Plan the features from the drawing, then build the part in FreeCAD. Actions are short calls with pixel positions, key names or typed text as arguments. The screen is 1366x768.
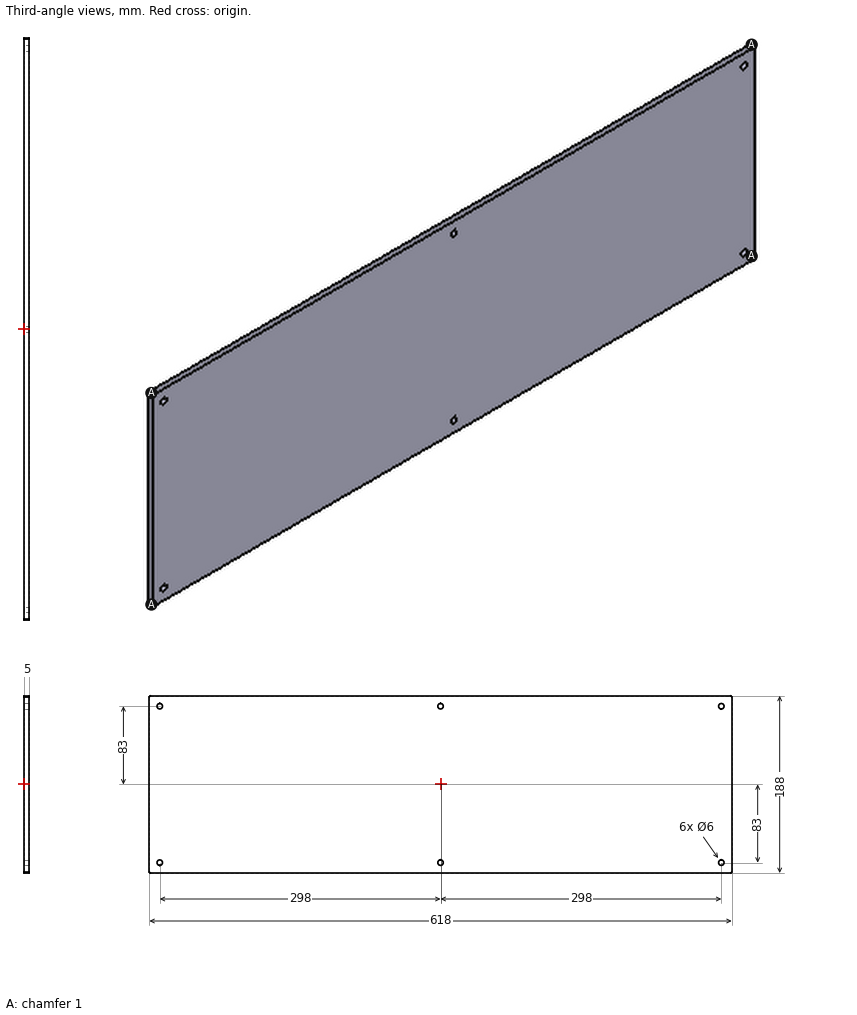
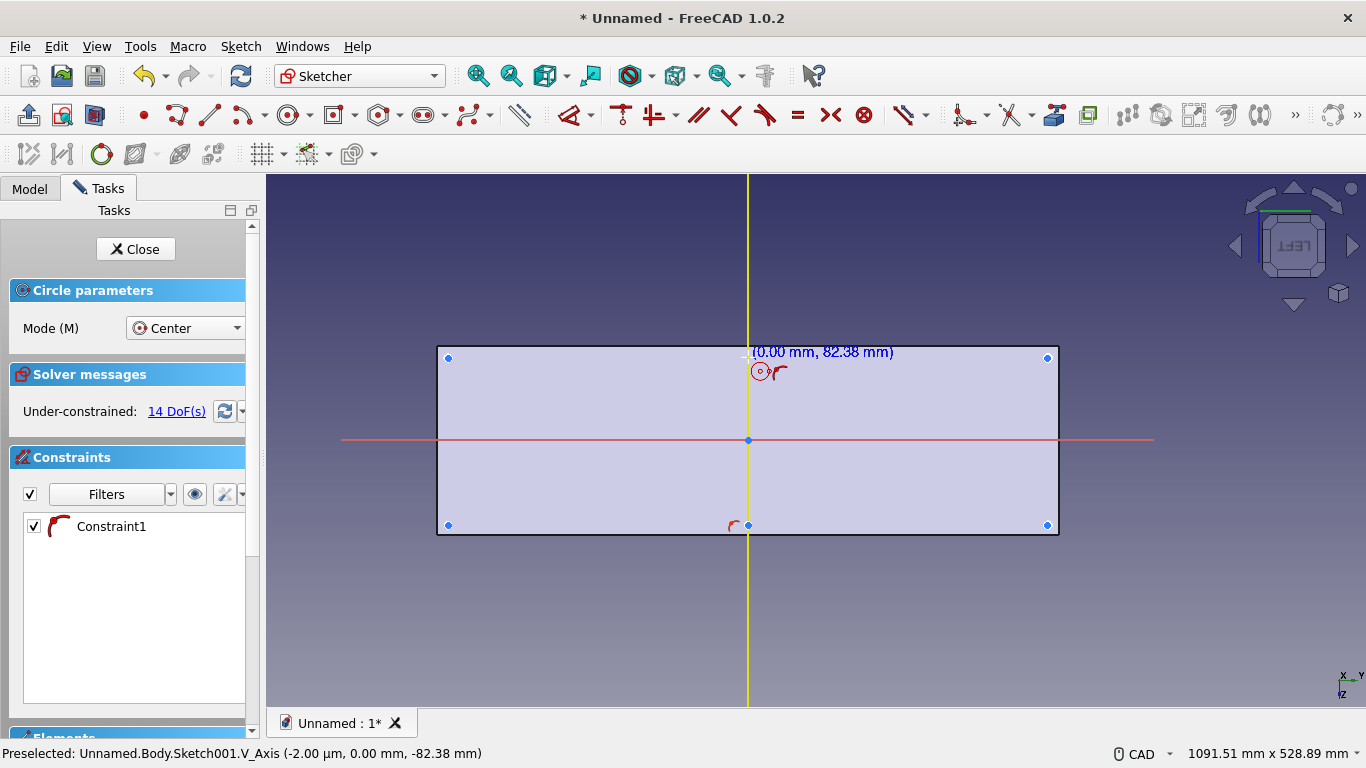
click(748, 357)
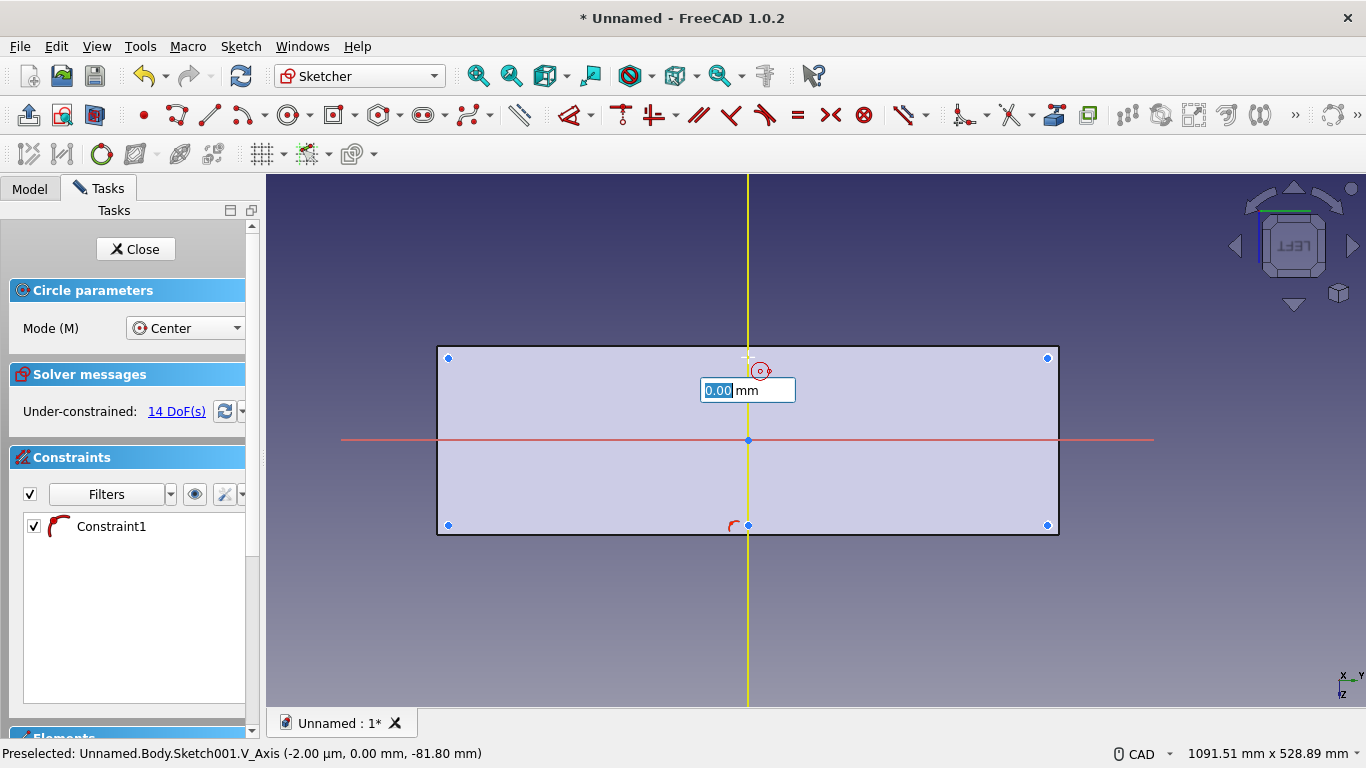
scroll(751, 356, up, 9)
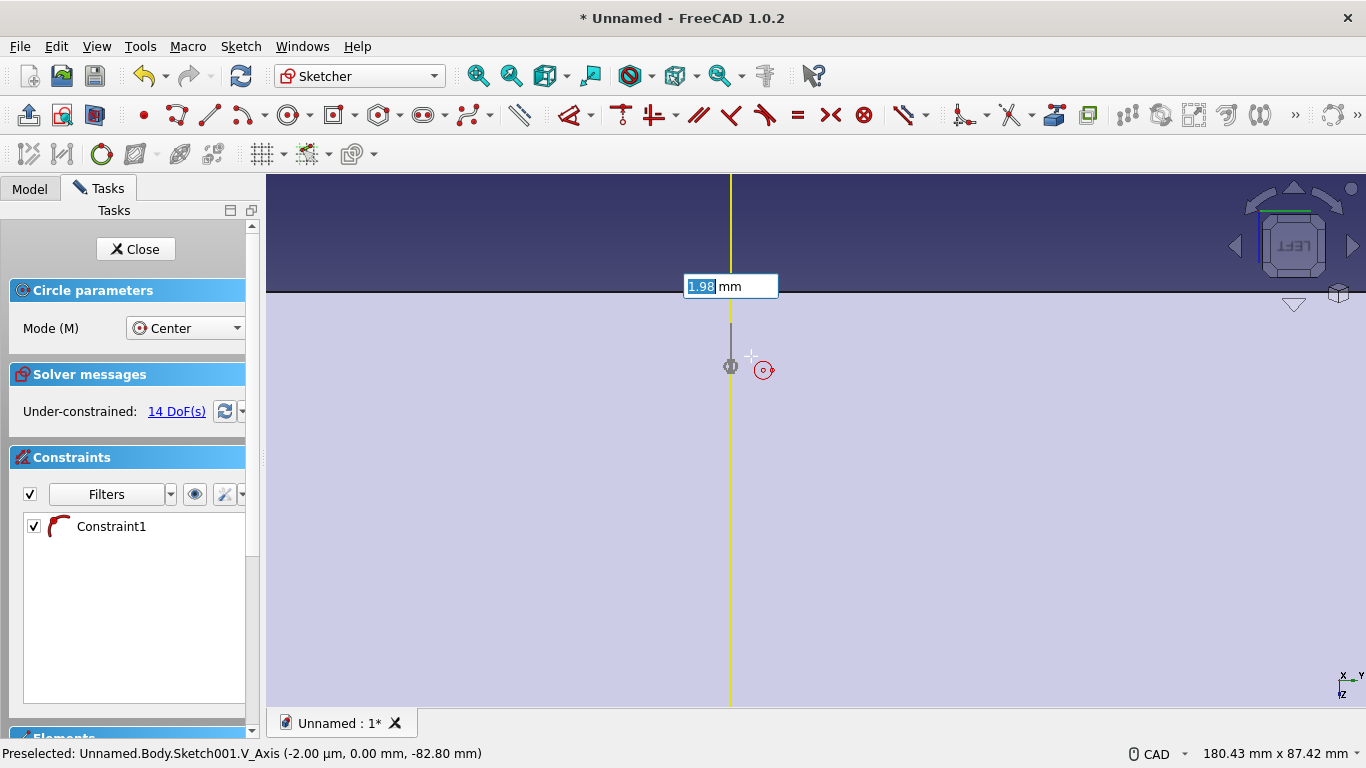
click(748, 353)
key(Escape)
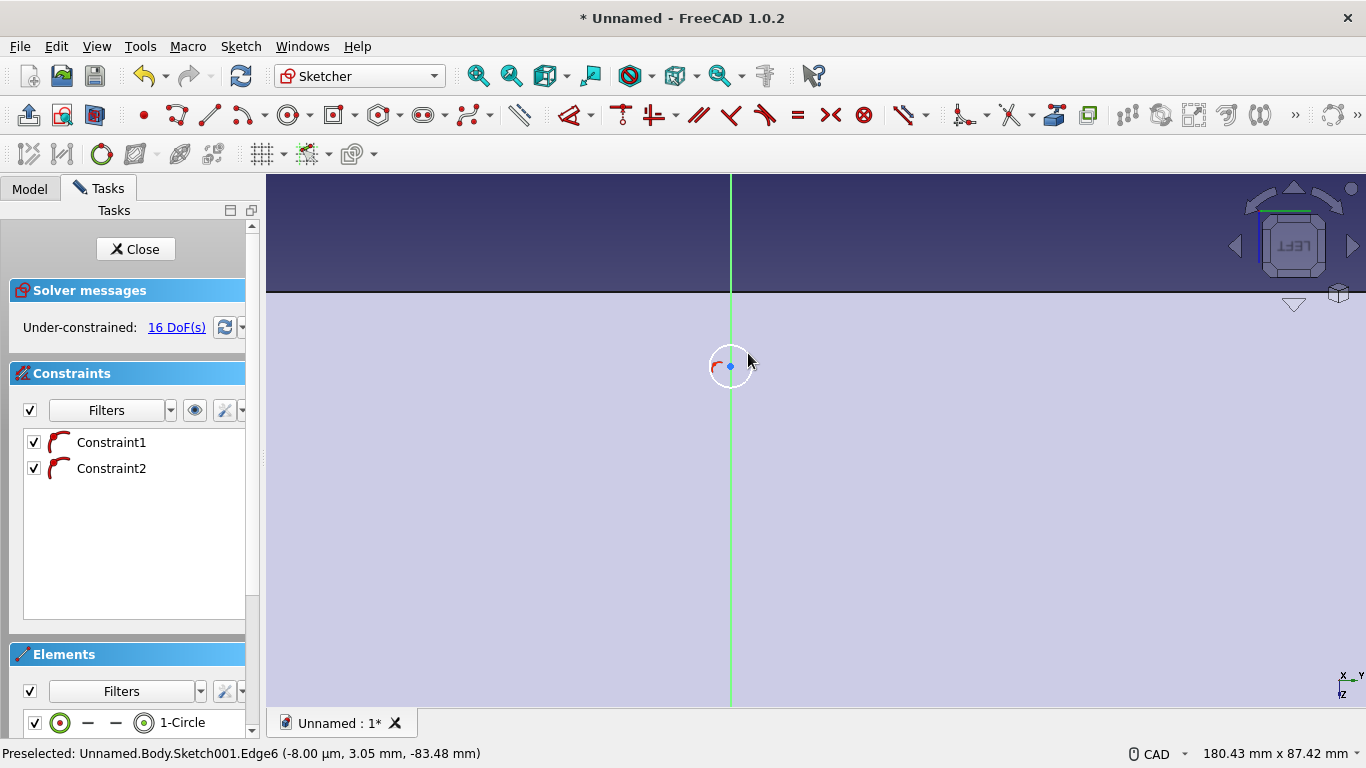
scroll(751, 356, down, 9)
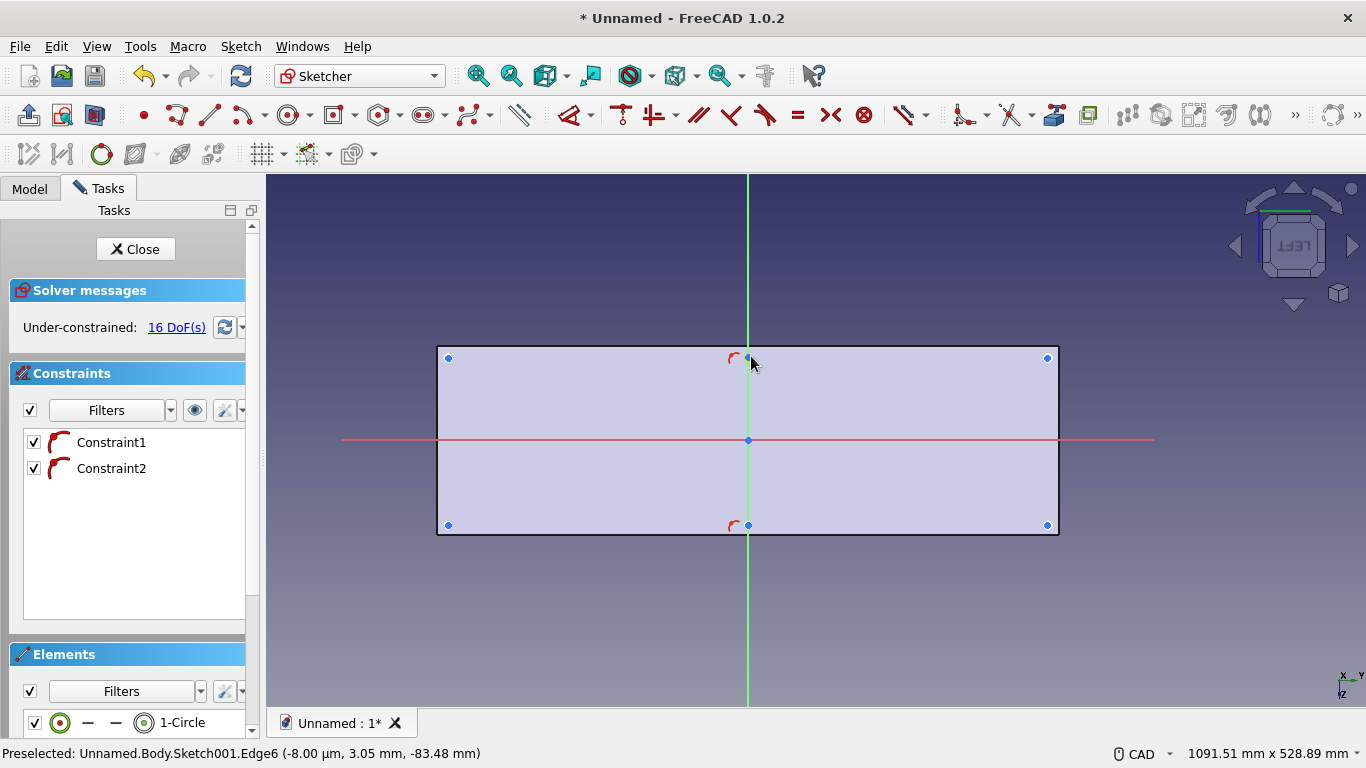
scroll(1051, 355, up, 7)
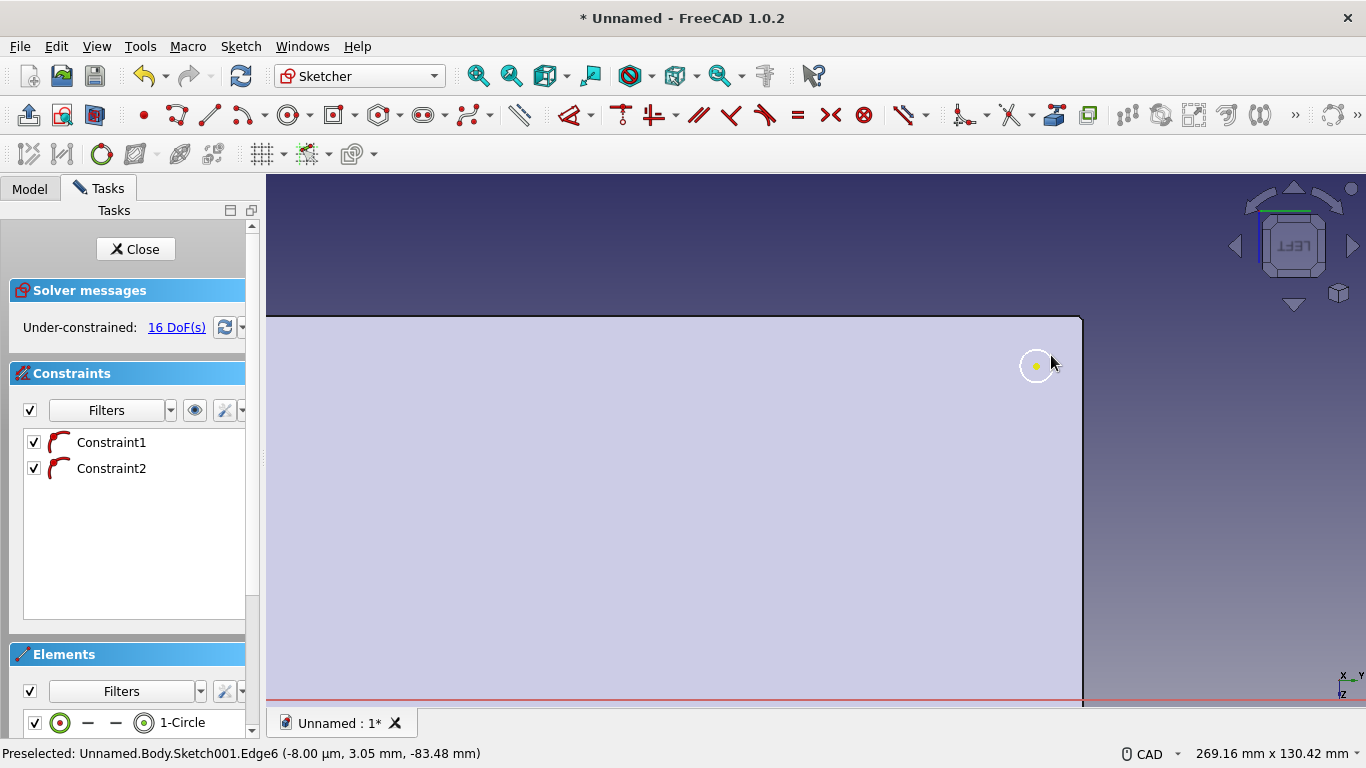
click(1048, 355)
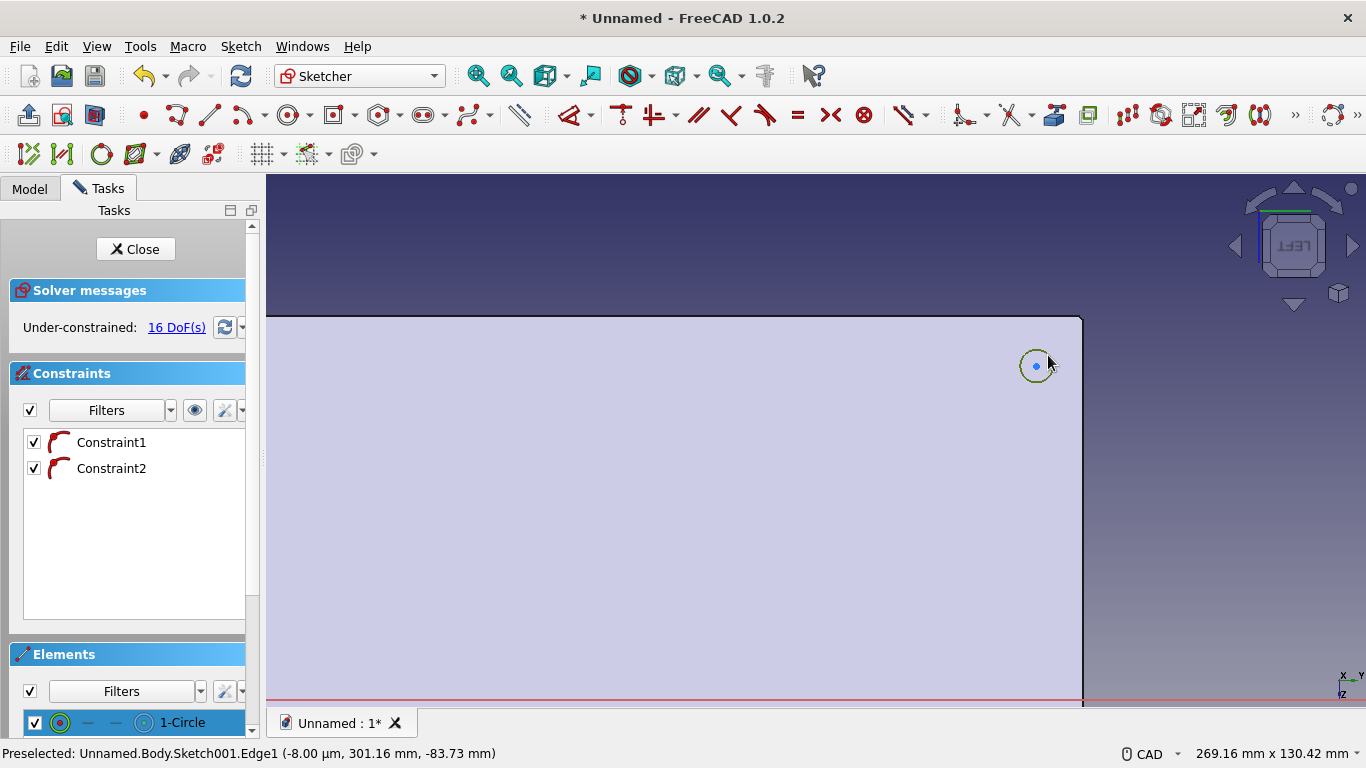
scroll(1051, 355, down, 7)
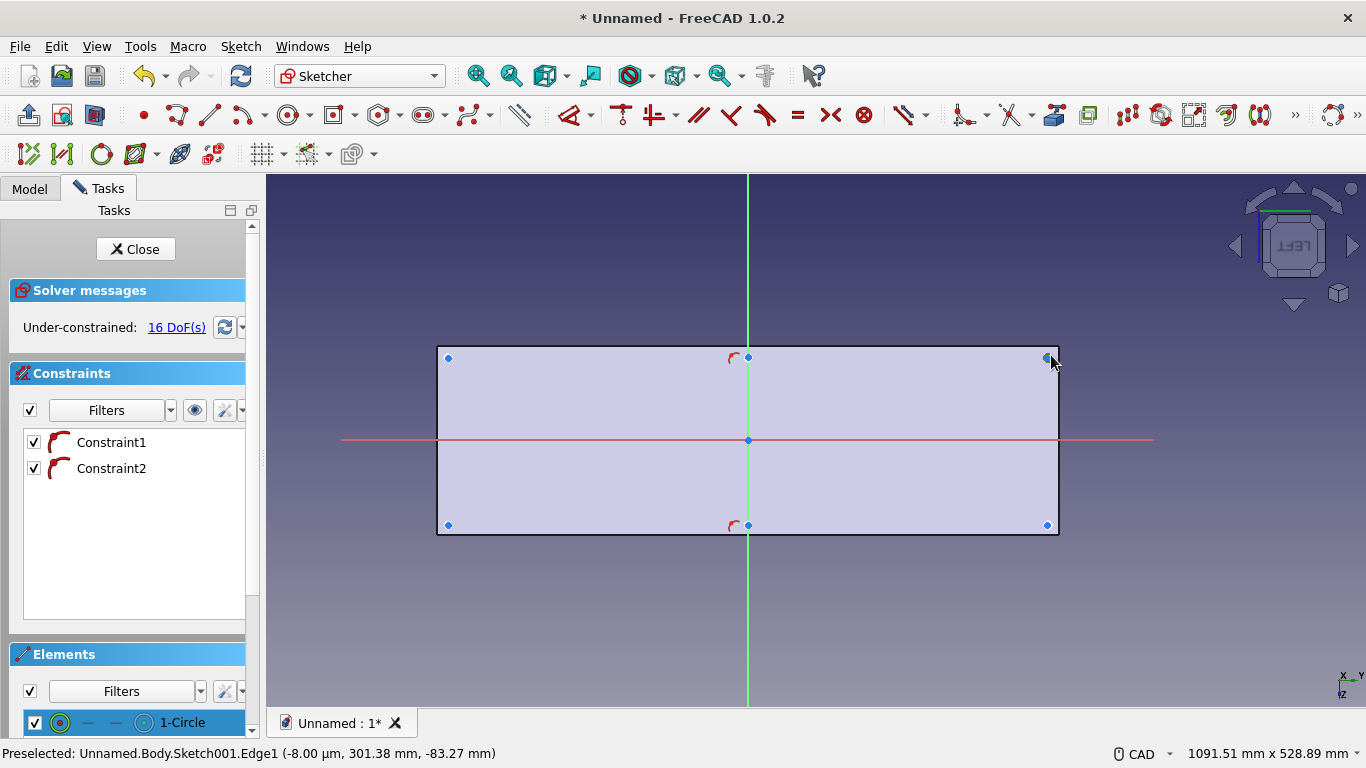
scroll(451, 355, up, 7)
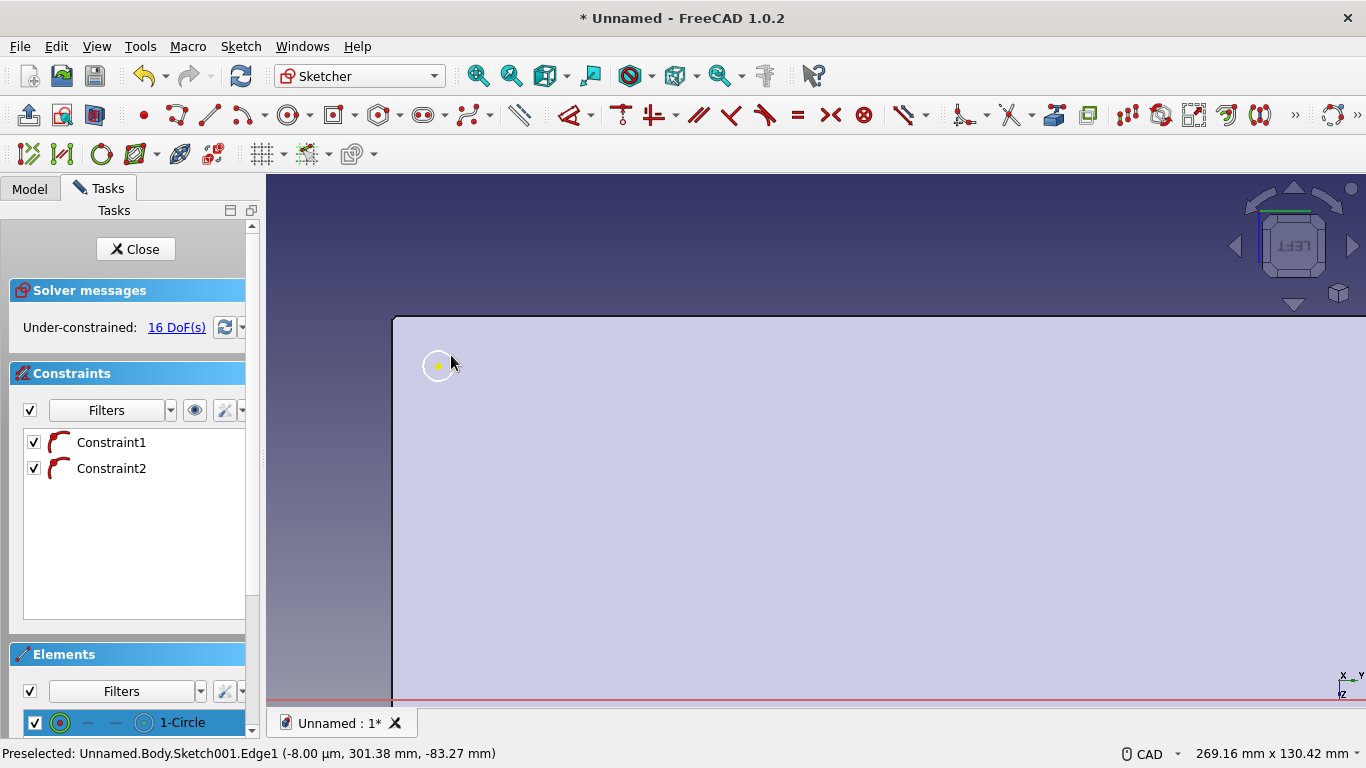
click(449, 356)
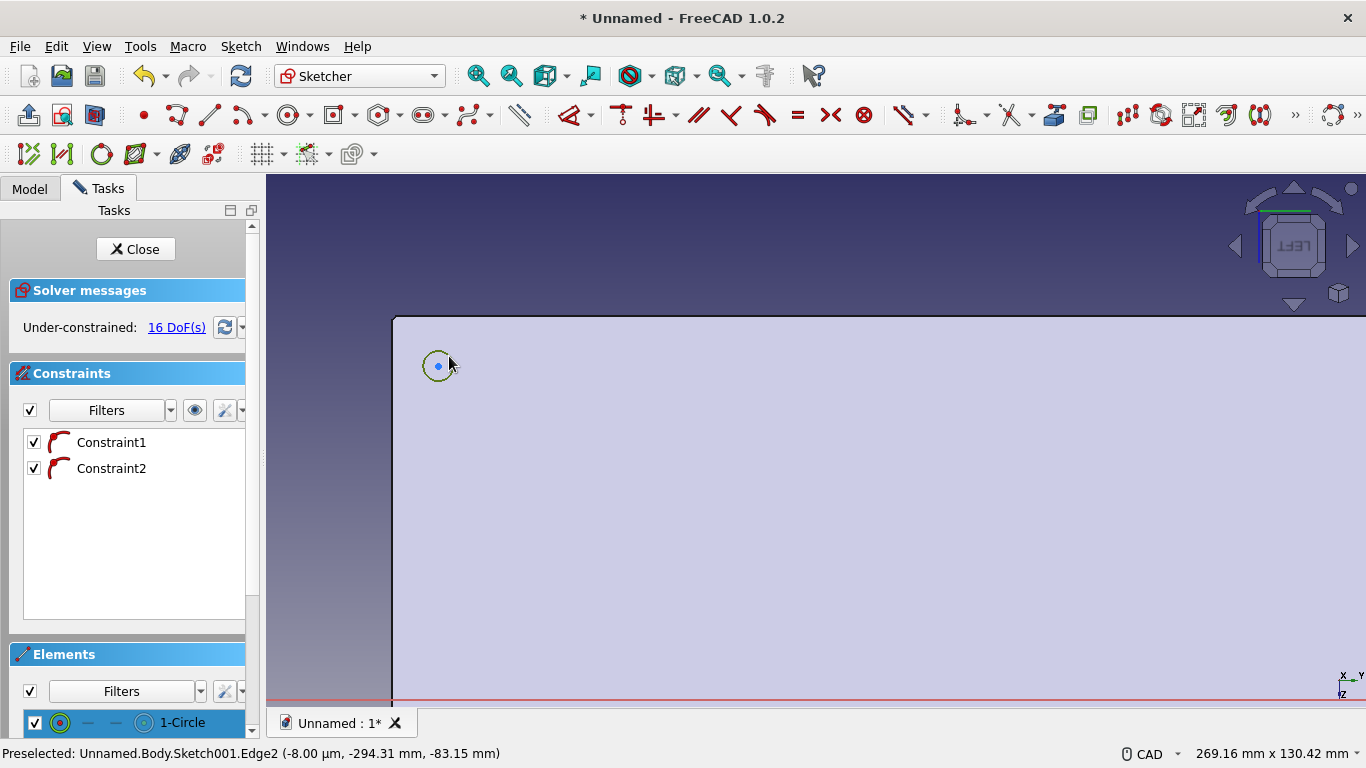
scroll(450, 355, down, 7)